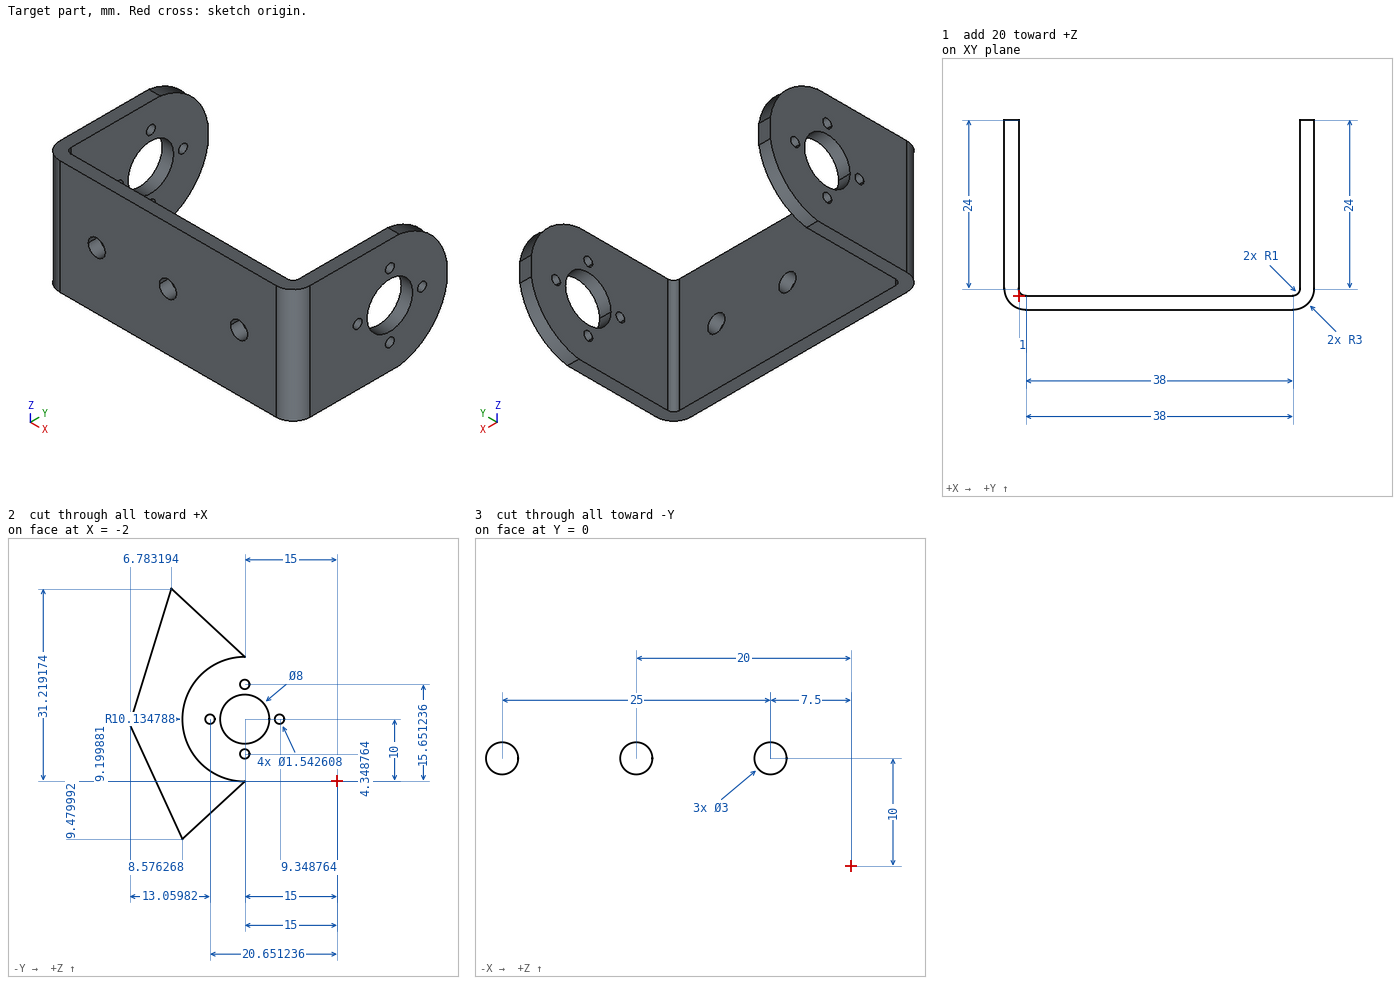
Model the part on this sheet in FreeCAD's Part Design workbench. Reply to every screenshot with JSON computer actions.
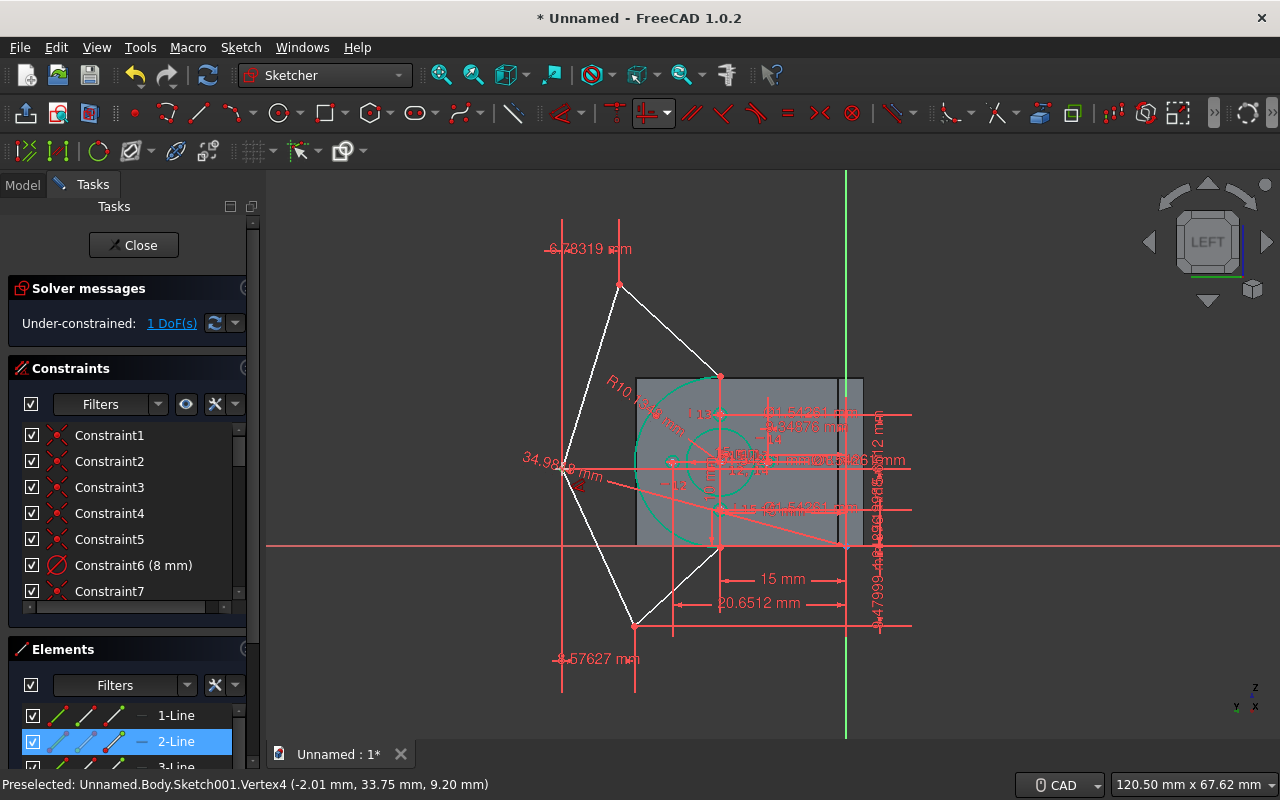
{"action": "left_click", "coordinate": [673, 462]}
{"action": "left_click", "coordinate": [618, 503]}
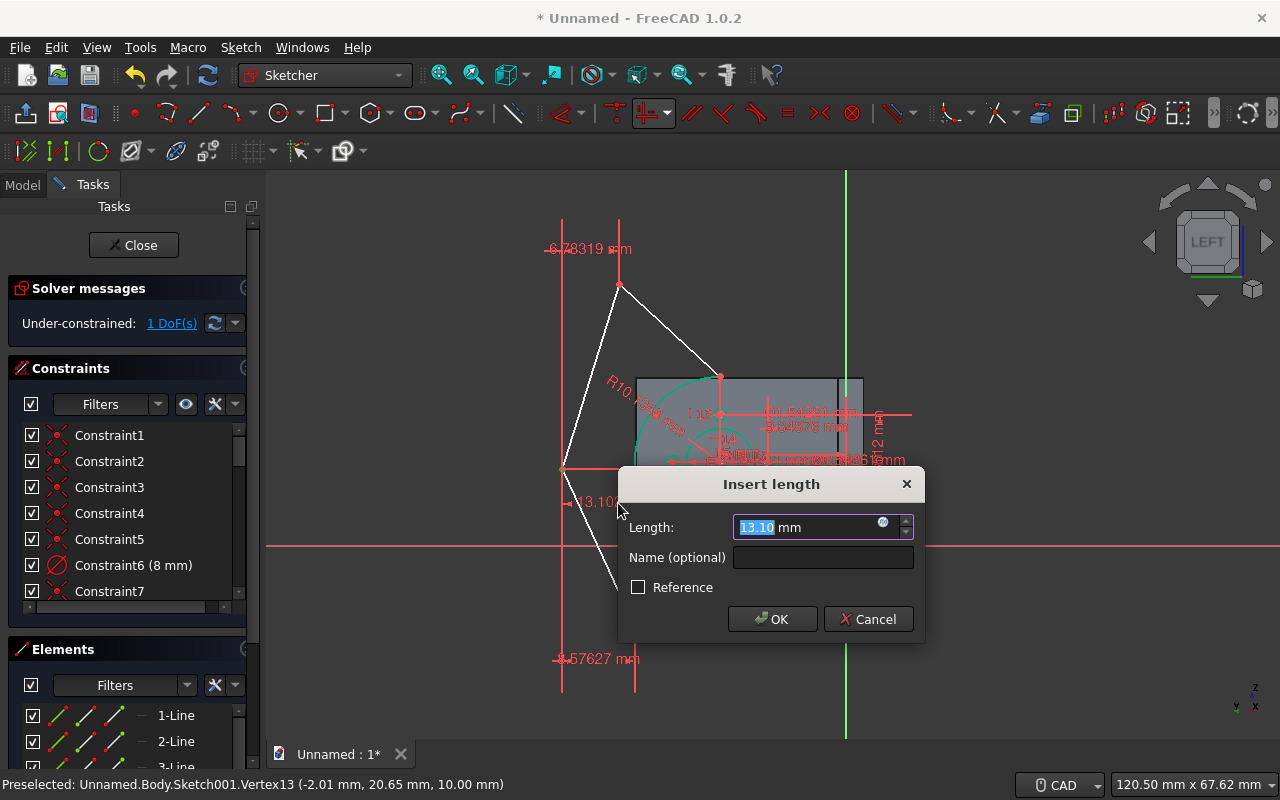
{"action": "type", "text": "13.05982"}
{"action": "key", "text": "Return"}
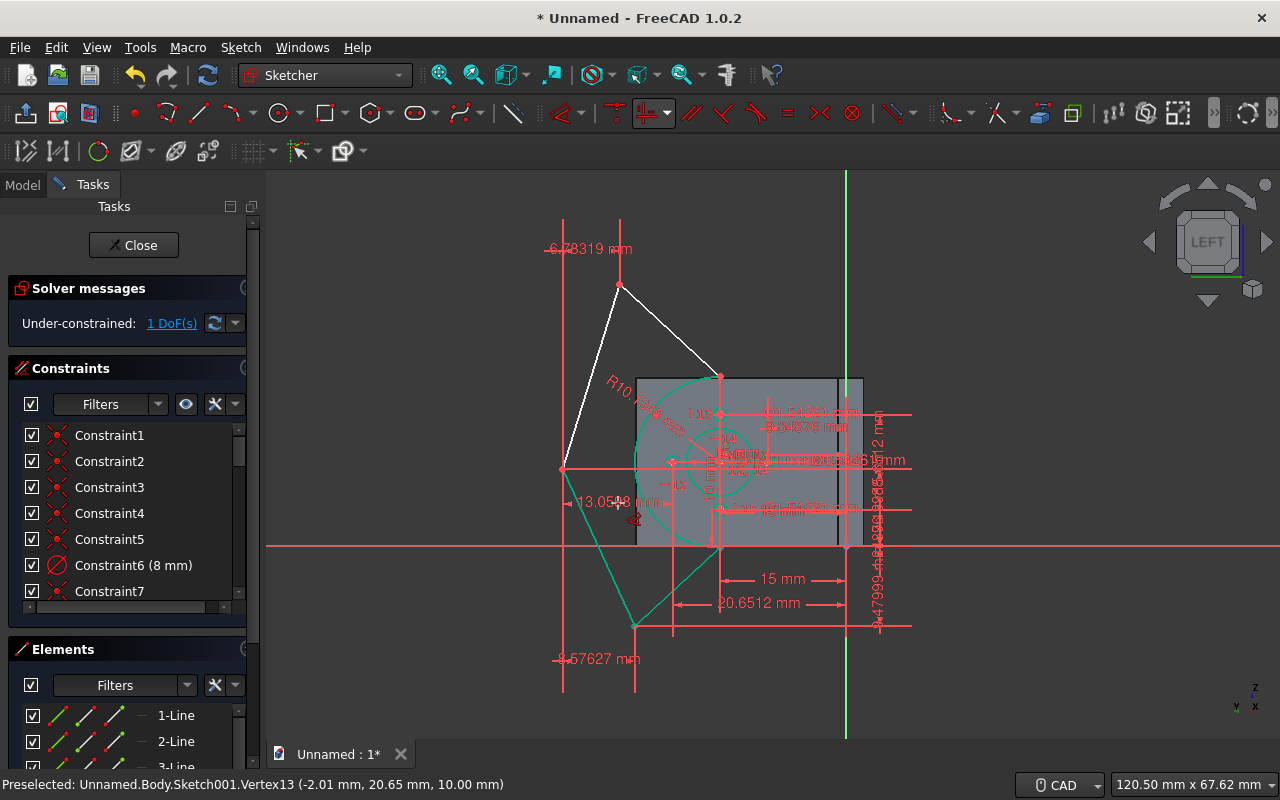
{"action": "left_click", "coordinate": [620, 284]}
{"action": "left_click", "coordinate": [880, 415]}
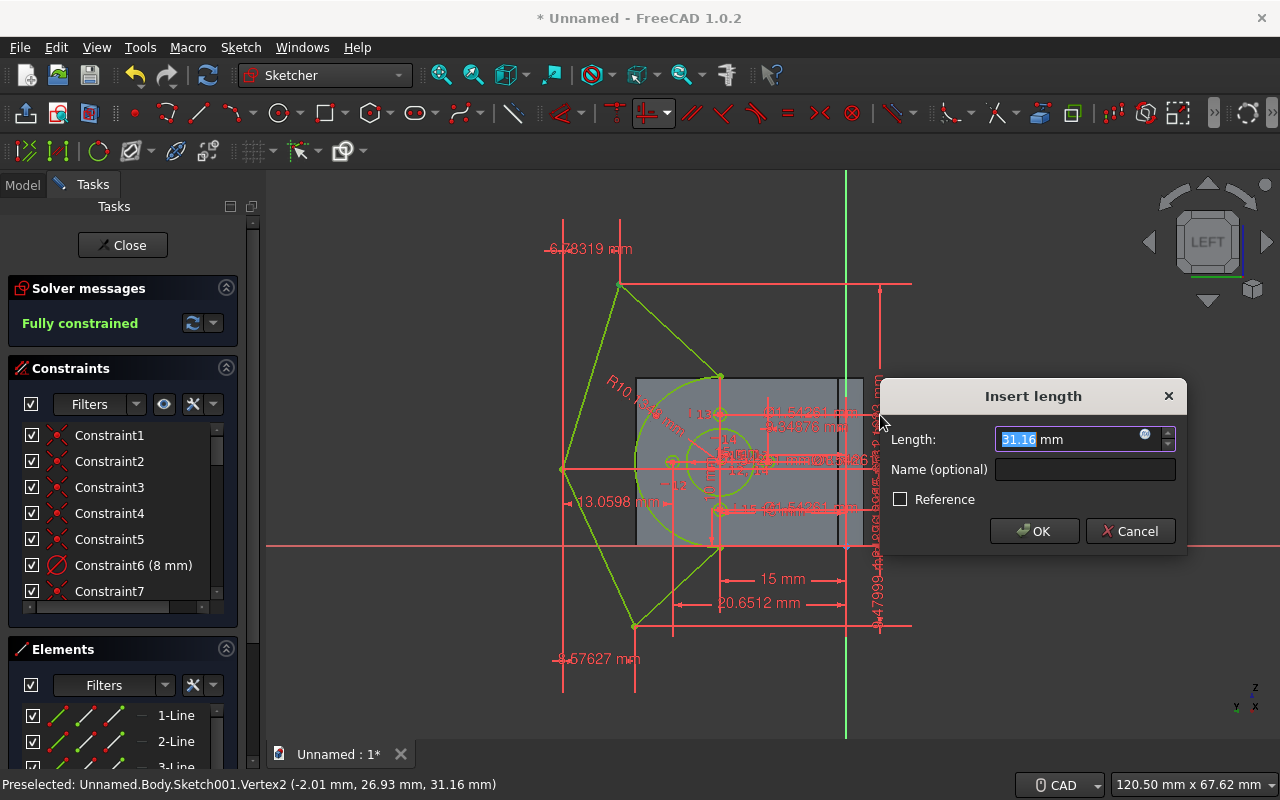
{"action": "type", "text": "31.219174"}
{"action": "key", "text": "Return"}
{"action": "key", "text": "Escape"}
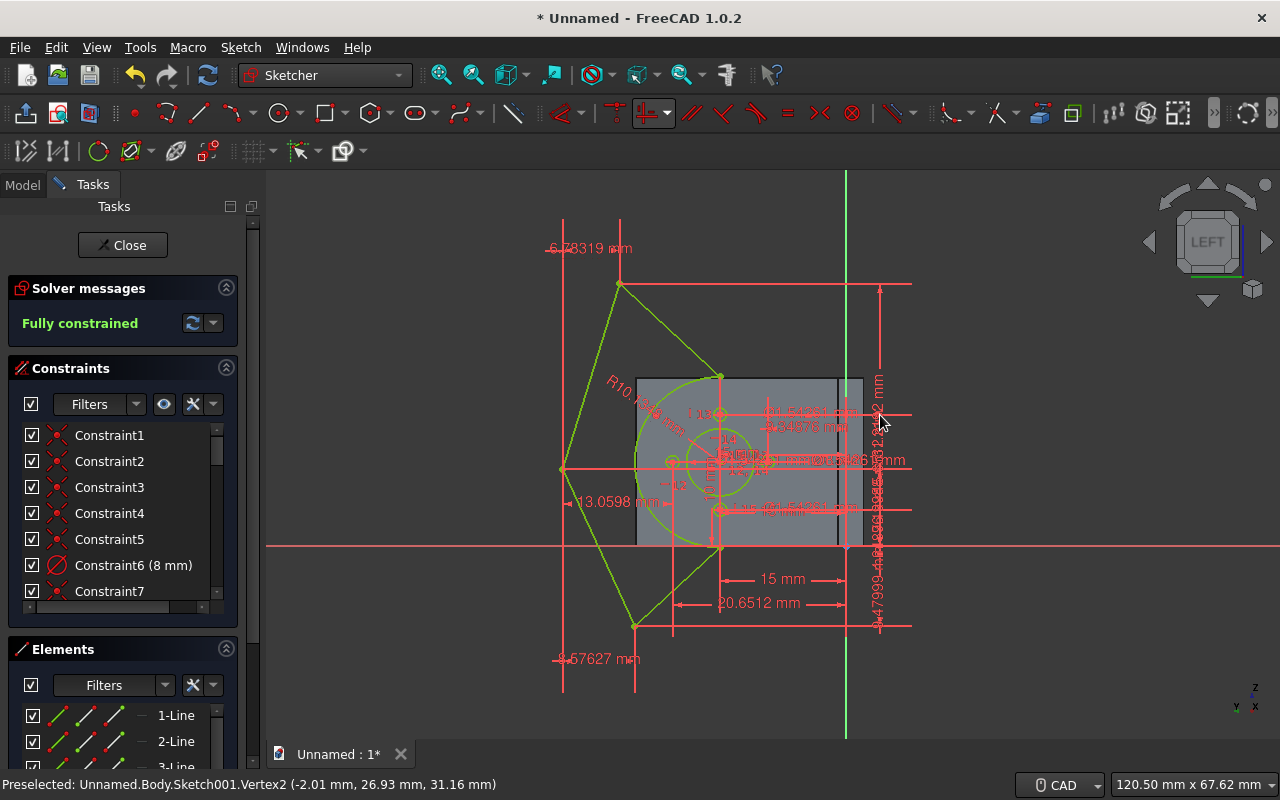
{"action": "left_click", "coordinate": [123, 245]}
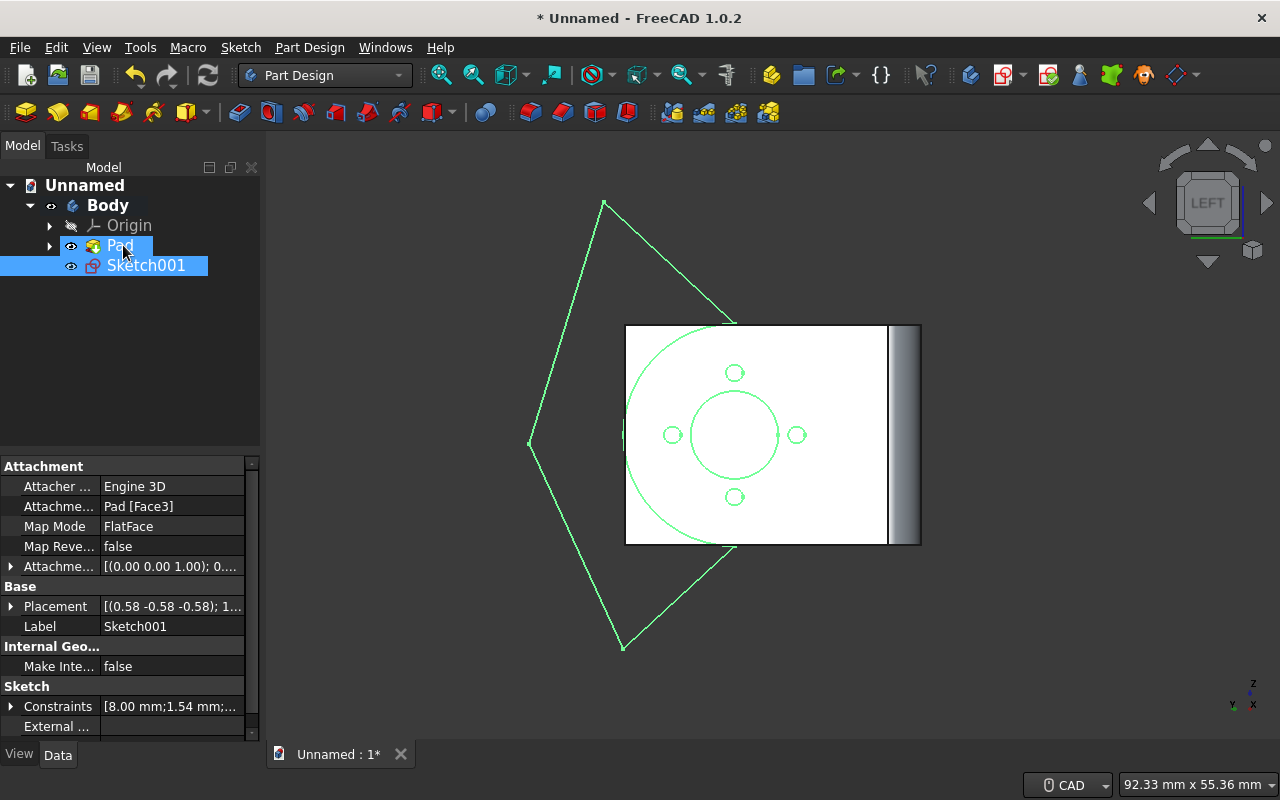
{"action": "left_click", "coordinate": [240, 112]}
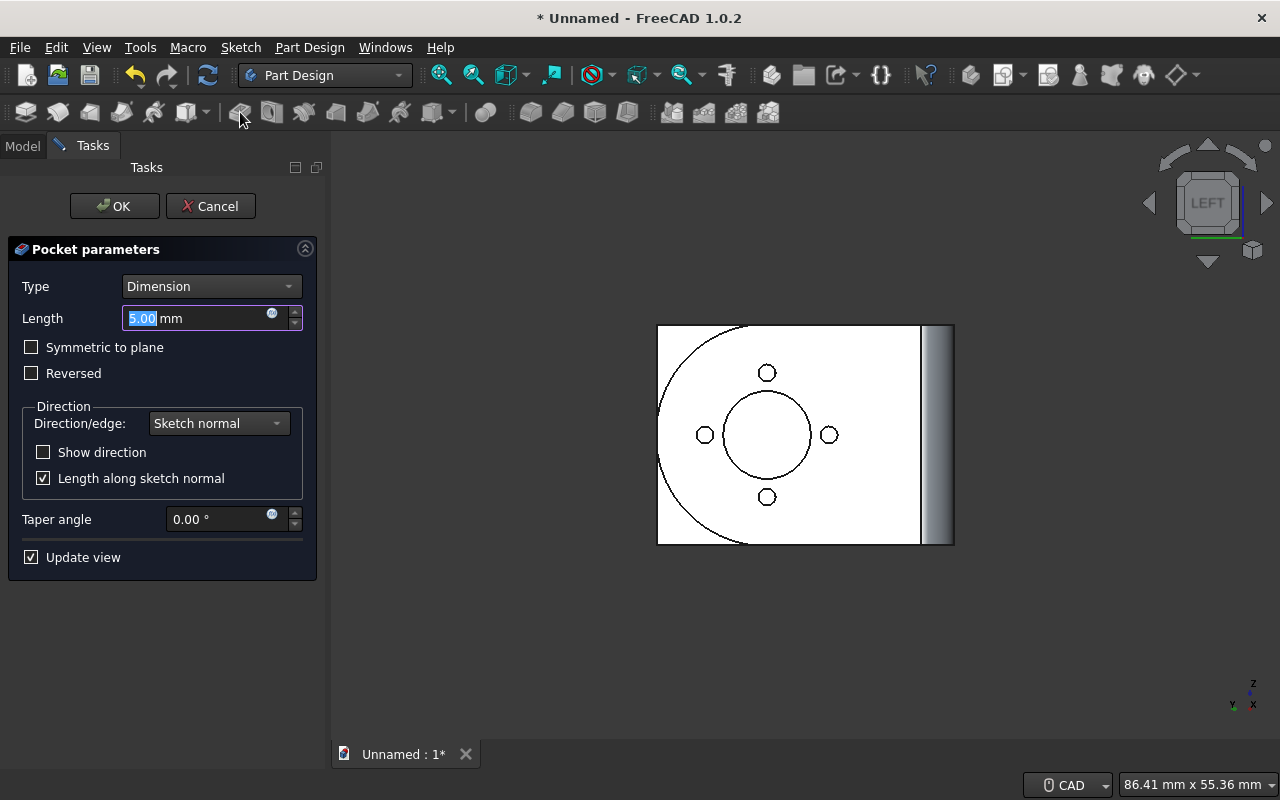
{"action": "left_click", "coordinate": [212, 286]}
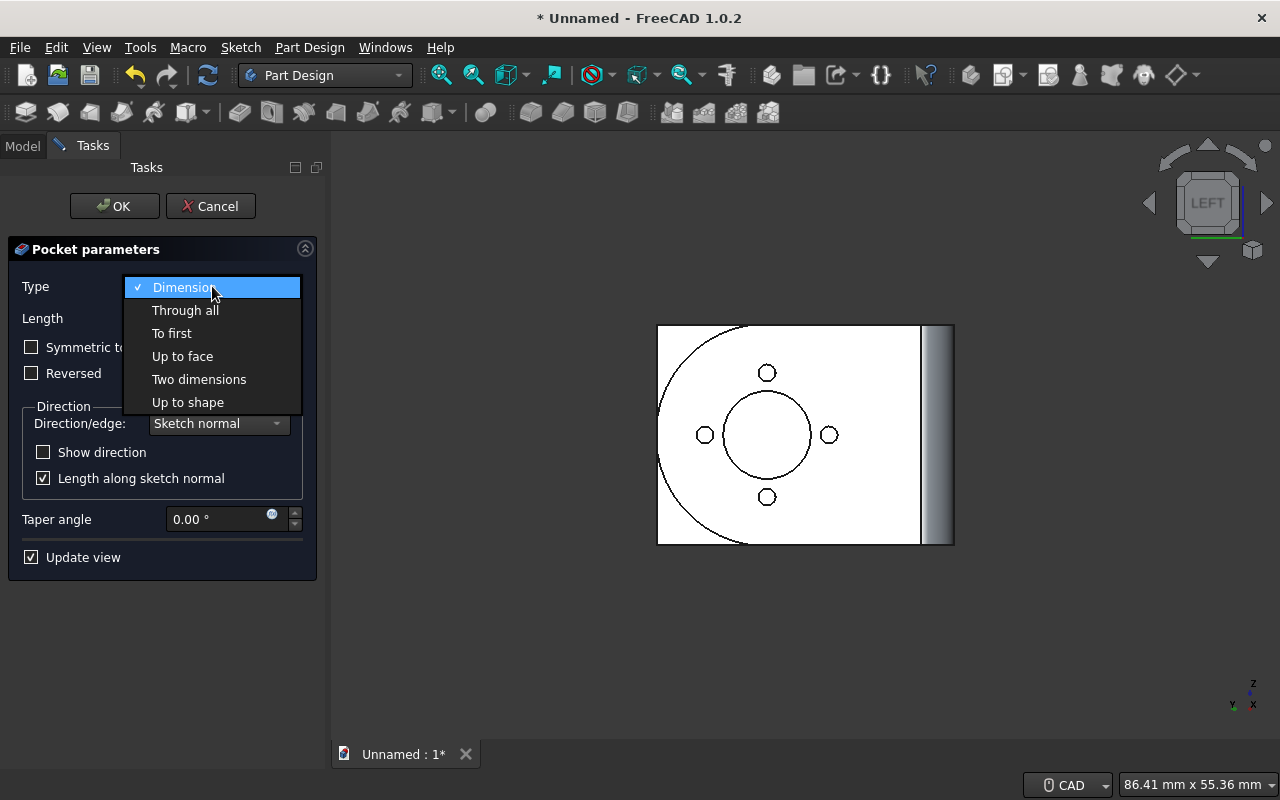
{"action": "left_click", "coordinate": [212, 310]}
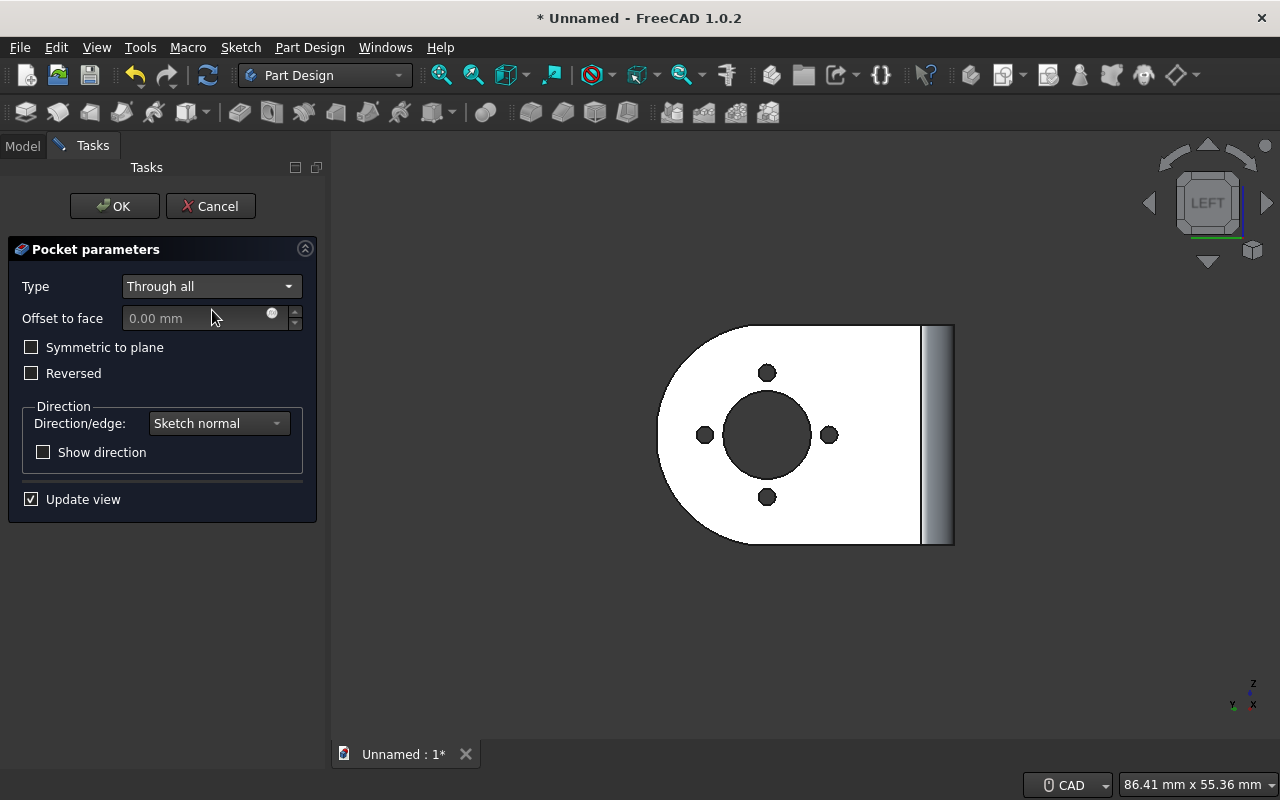
{"action": "left_click", "coordinate": [115, 206]}